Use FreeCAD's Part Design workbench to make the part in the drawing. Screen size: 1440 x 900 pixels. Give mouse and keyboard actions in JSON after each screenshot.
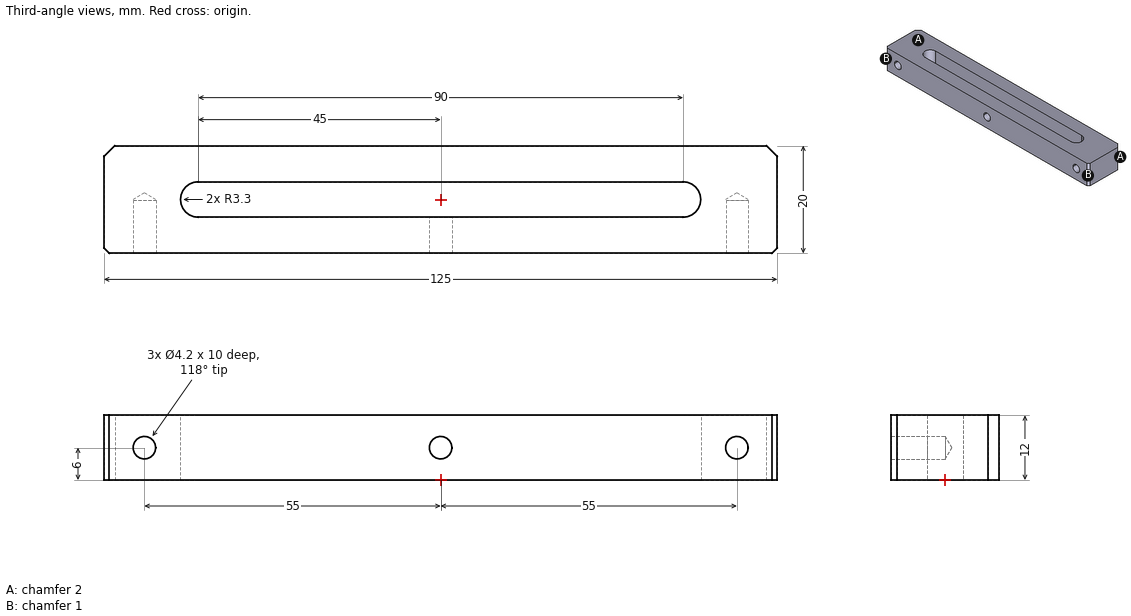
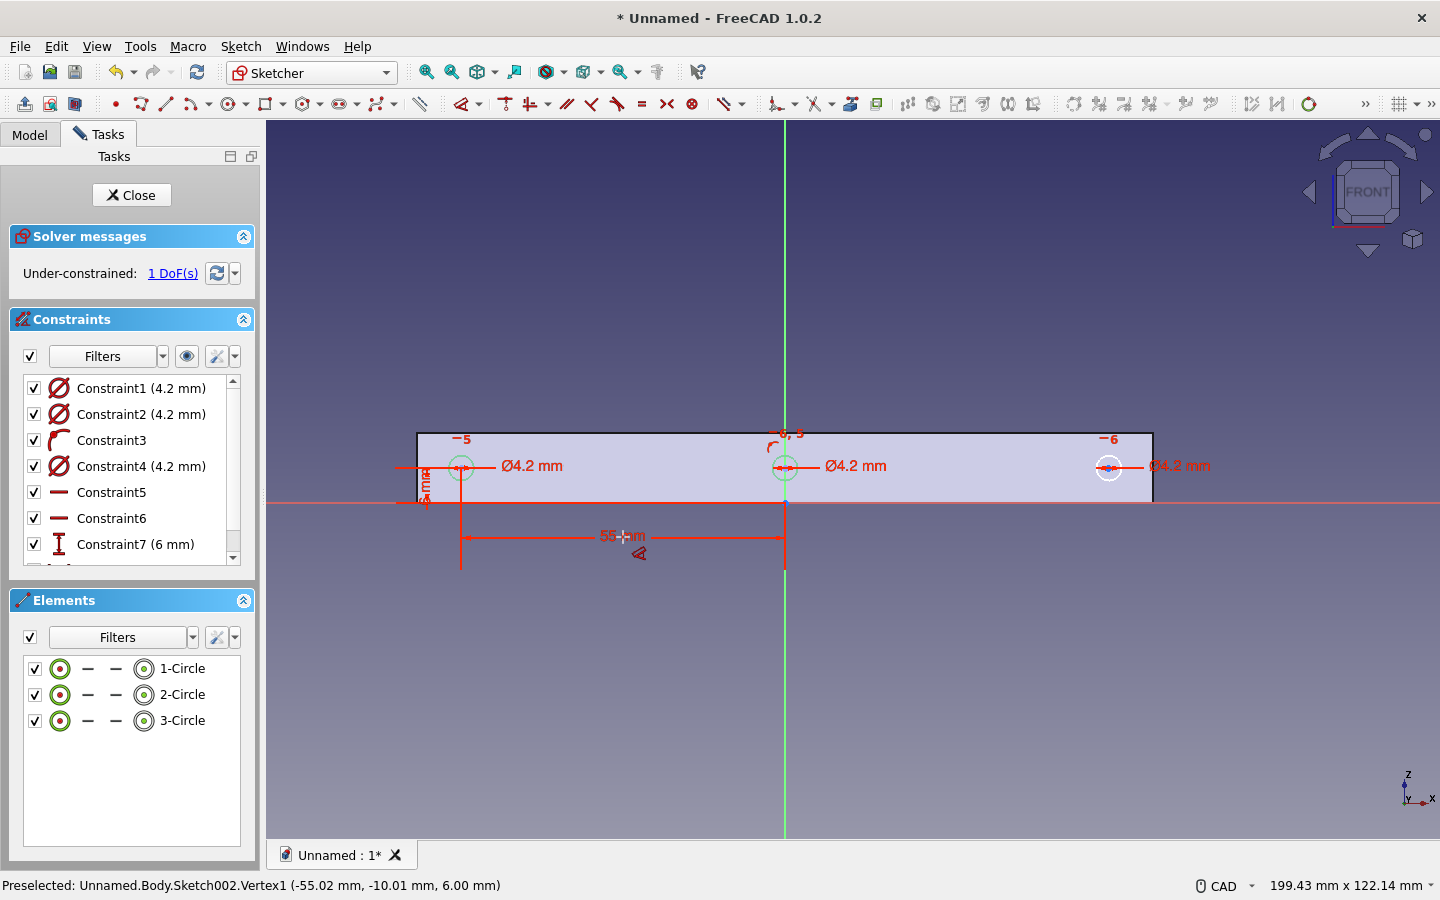
{"action": "left_click", "coordinate": [1109, 468]}
{"action": "left_click", "coordinate": [947, 537]}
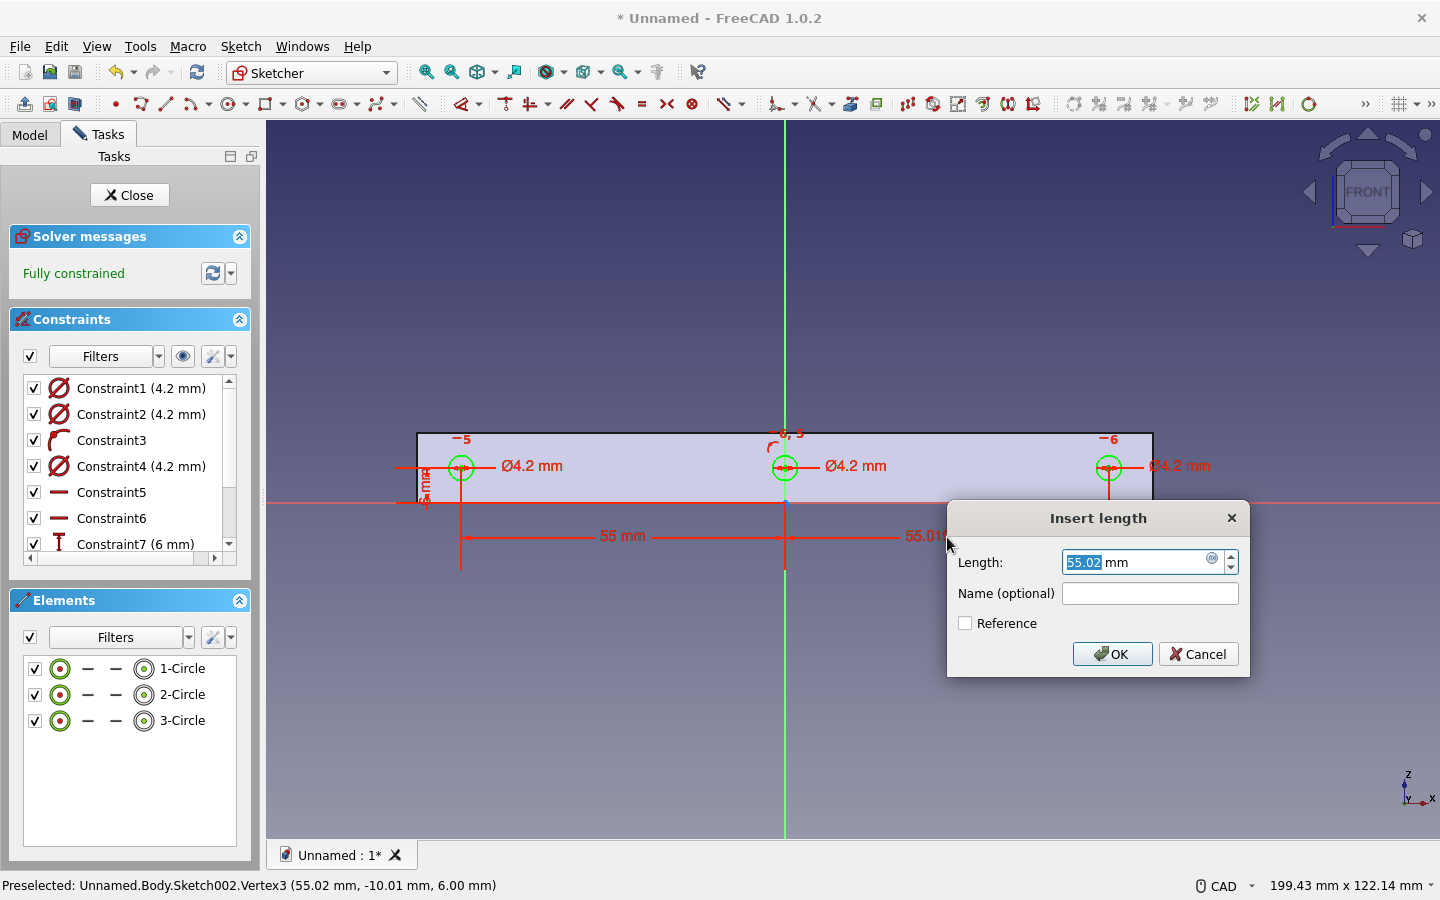
{"action": "type", "text": "55"}
{"action": "key", "text": "Return"}
{"action": "key", "text": "Escape"}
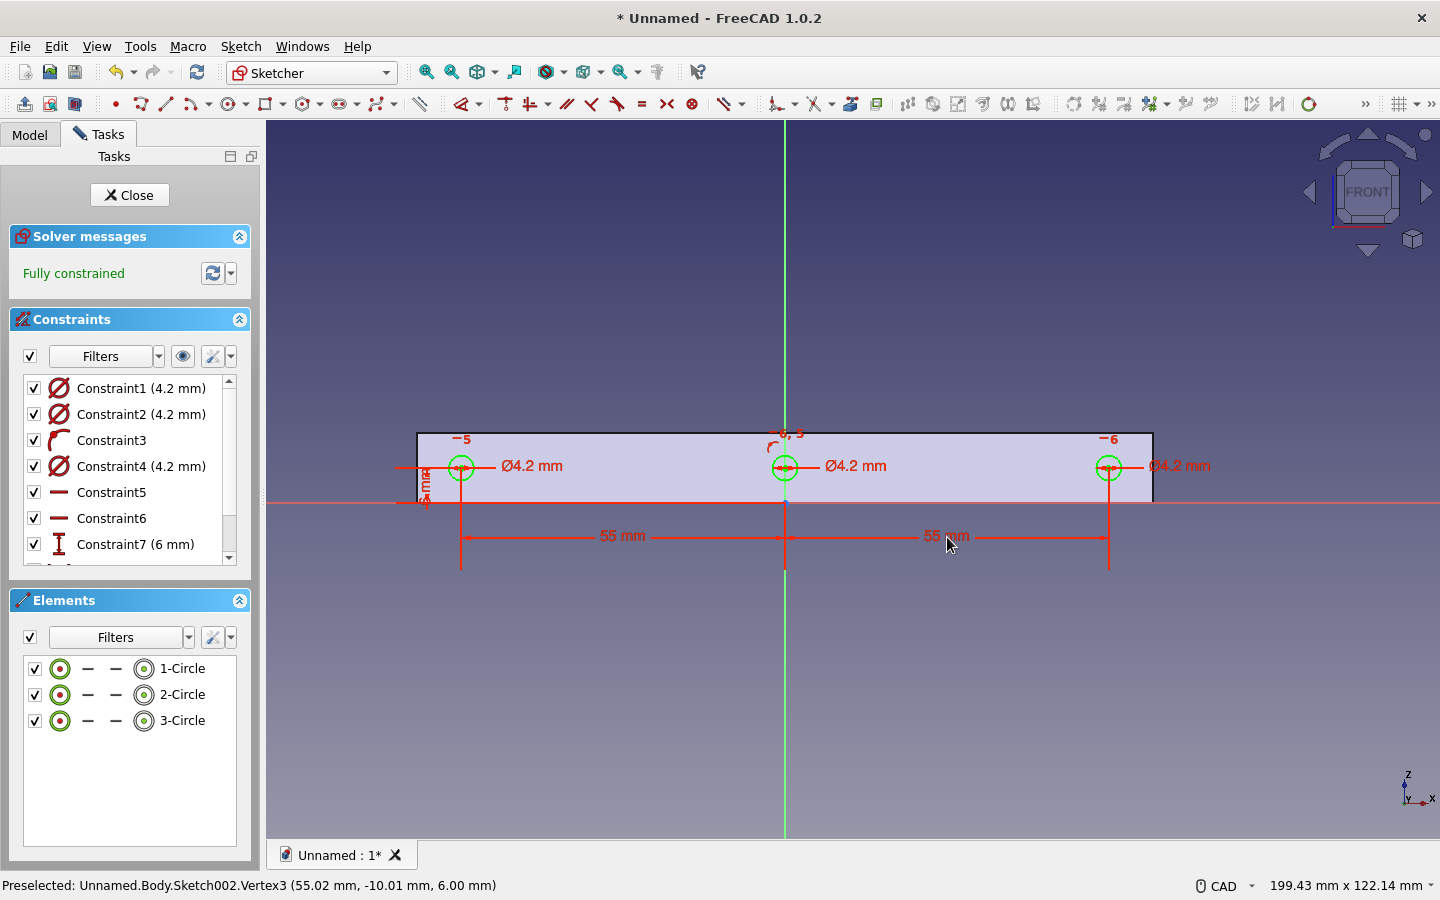
{"action": "left_click", "coordinate": [130, 195]}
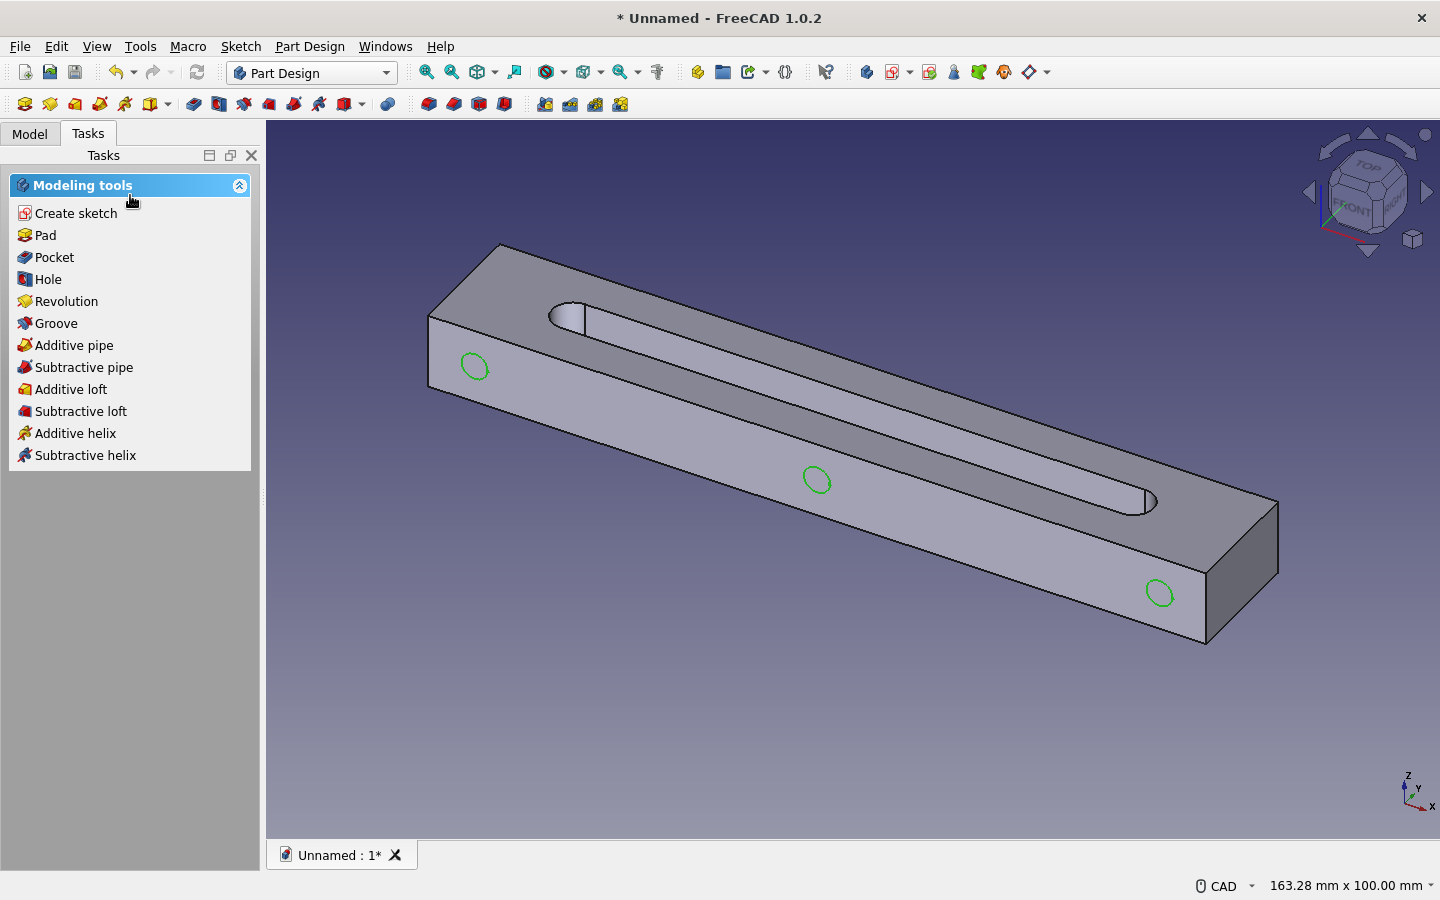
{"action": "left_click", "coordinate": [219, 104]}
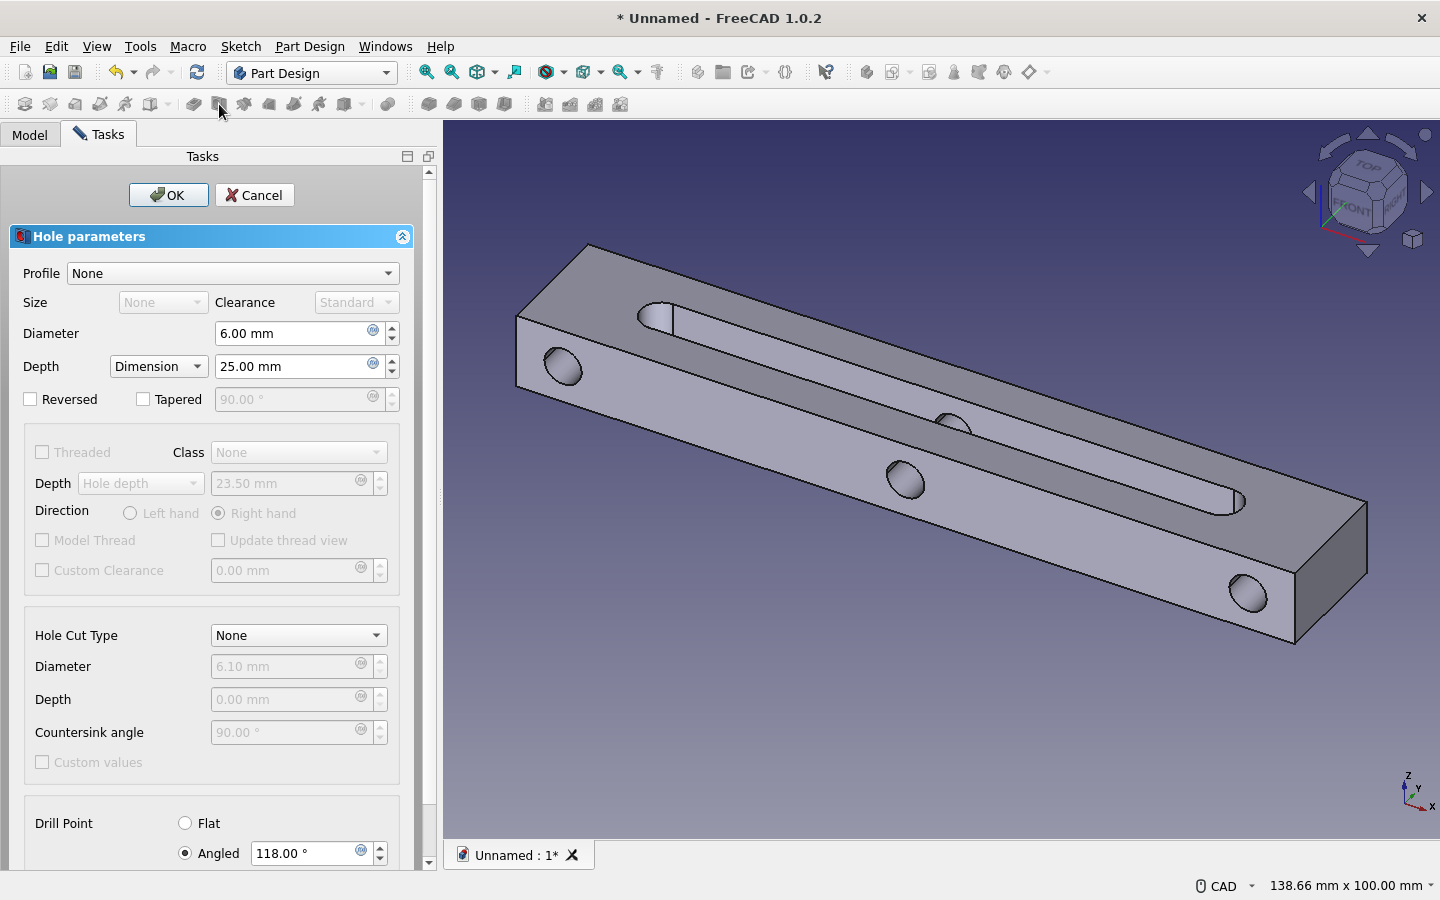
{"action": "triple_click", "coordinate": [300, 334]}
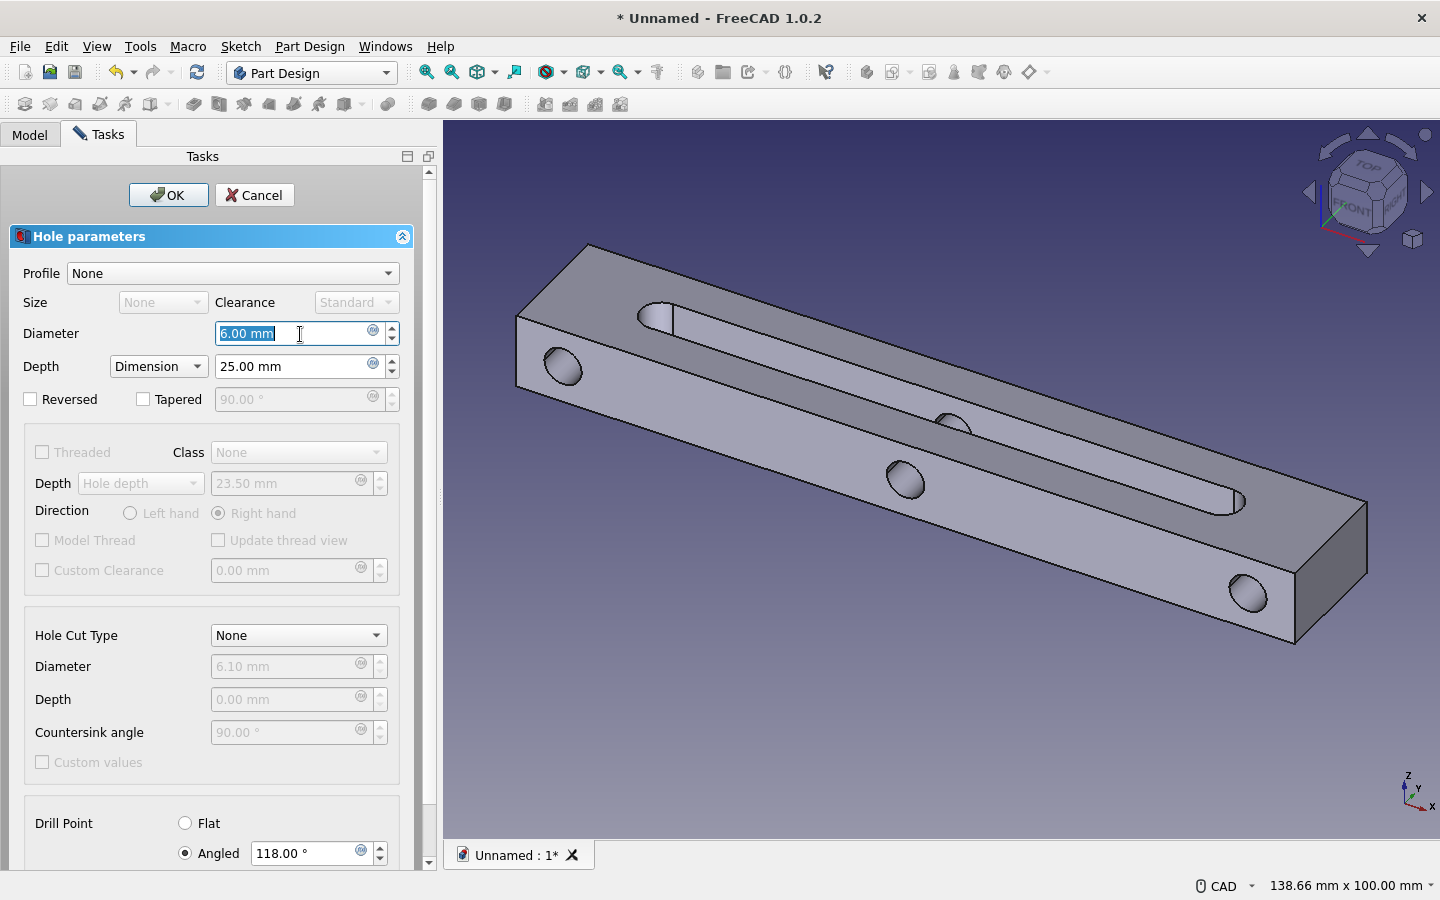
{"action": "type", "text": "4.2"}
{"action": "key", "text": "Tab"}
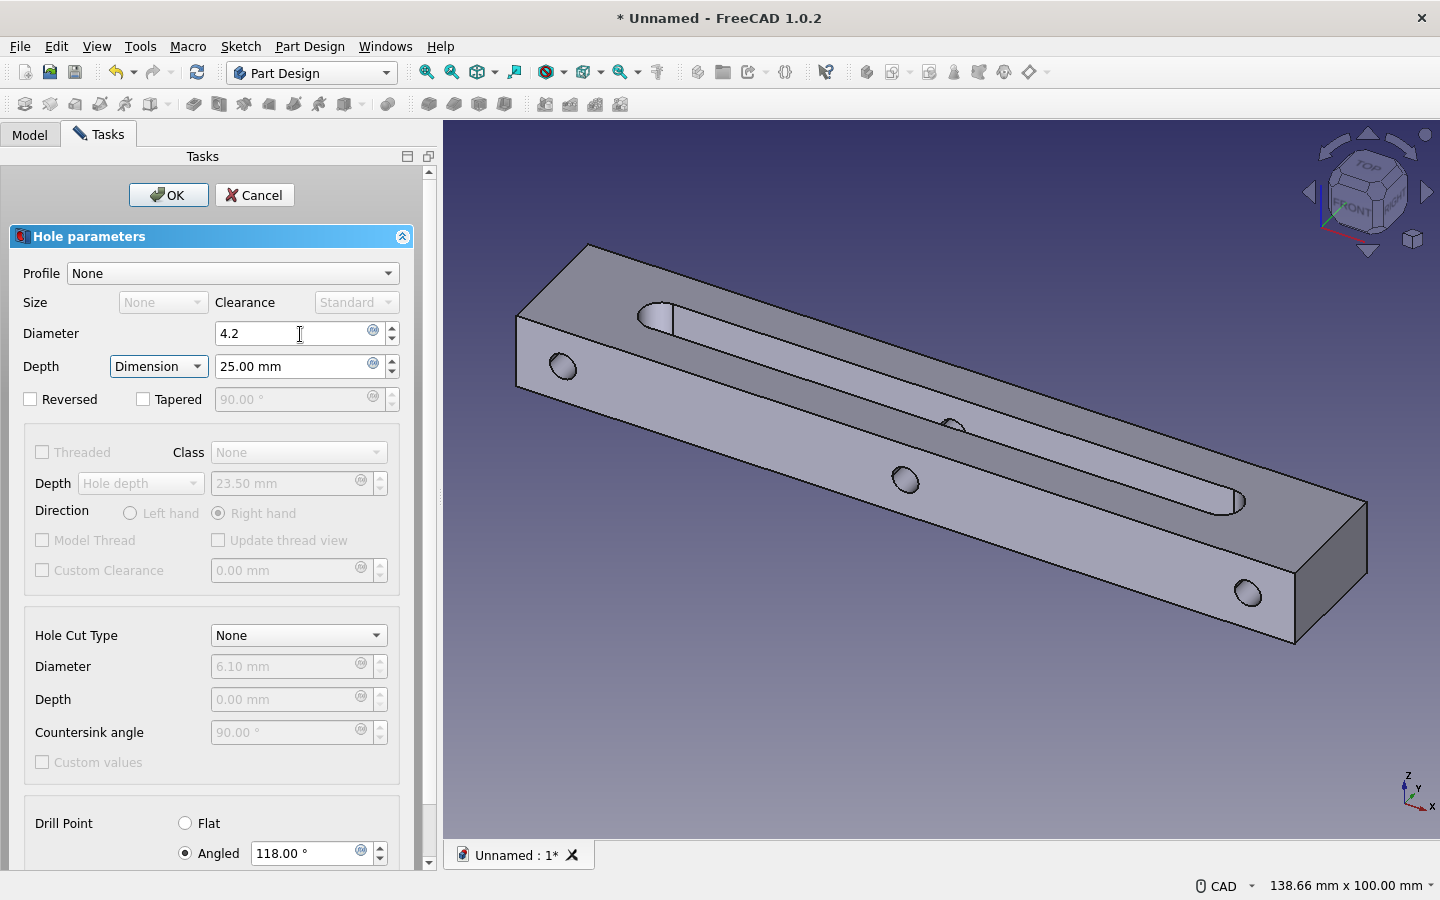
{"action": "triple_click", "coordinate": [300, 366]}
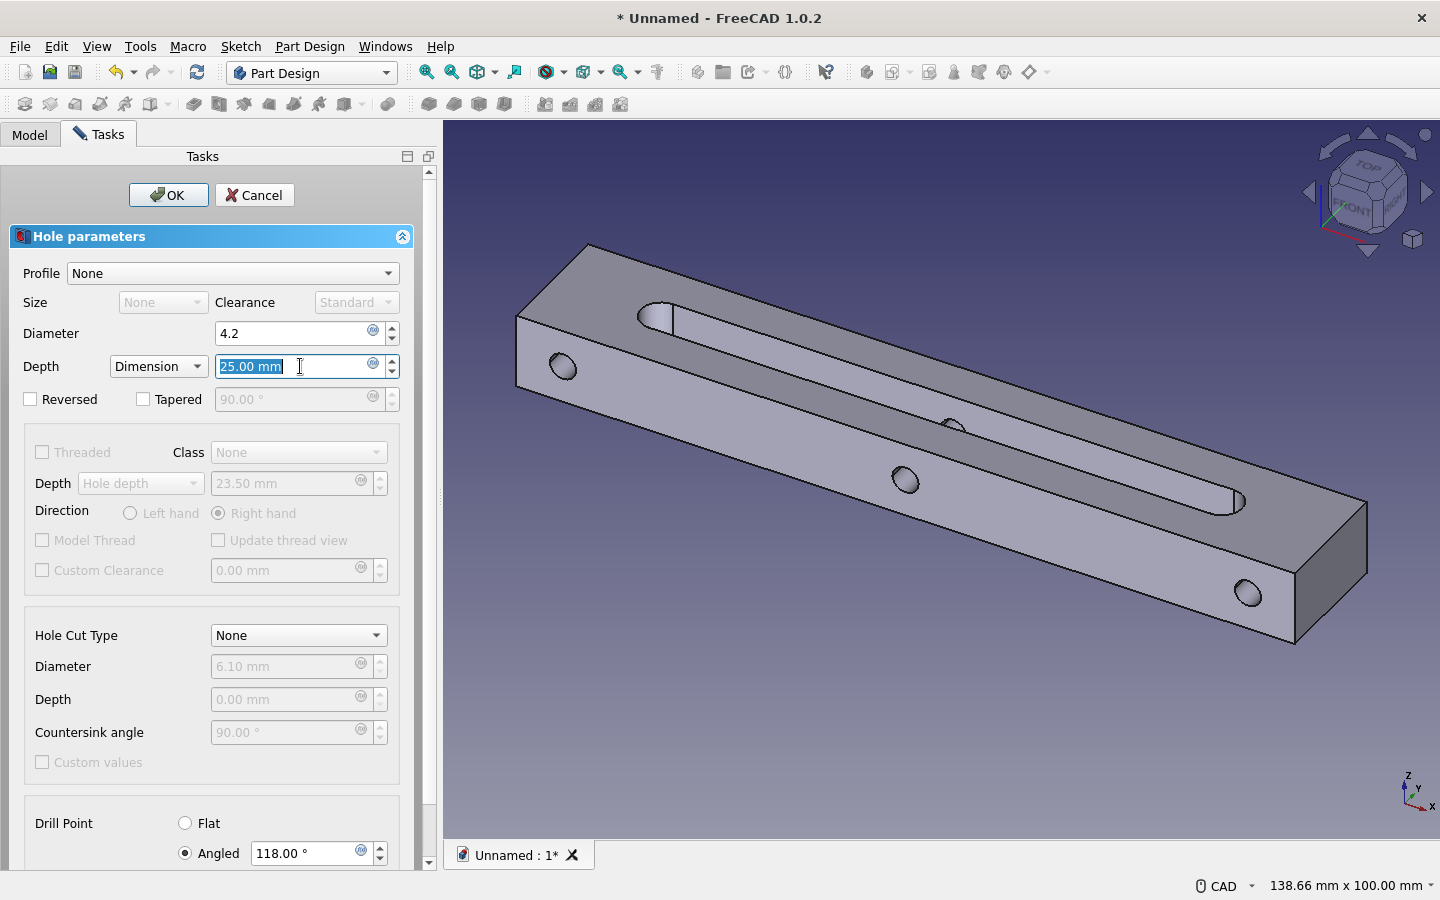
{"action": "type", "text": "10"}
{"action": "key", "text": "Tab"}